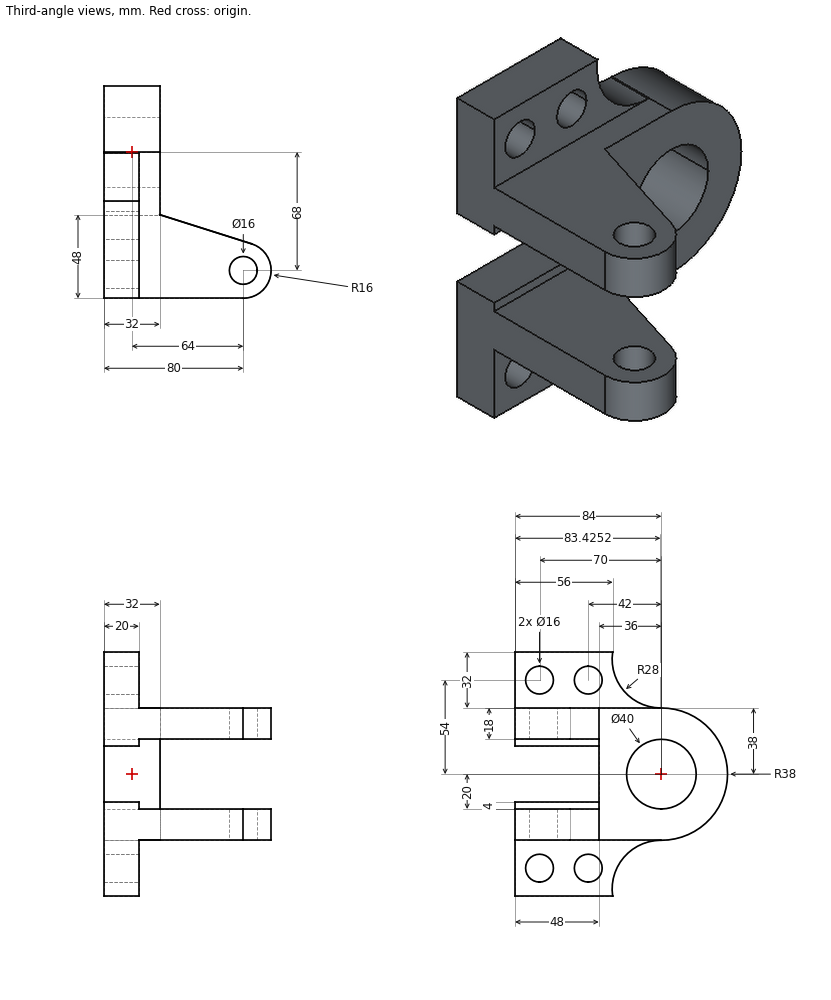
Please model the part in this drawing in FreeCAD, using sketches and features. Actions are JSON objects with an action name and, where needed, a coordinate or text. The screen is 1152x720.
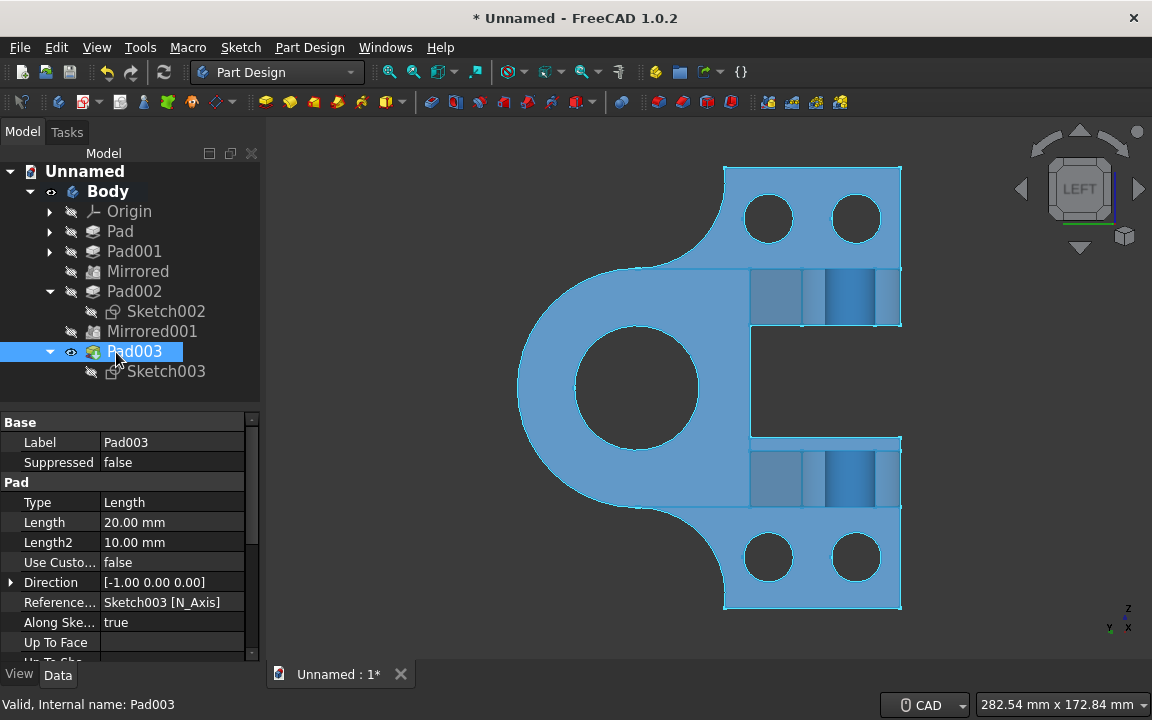
{"action": "left_click", "coordinate": [768, 102]}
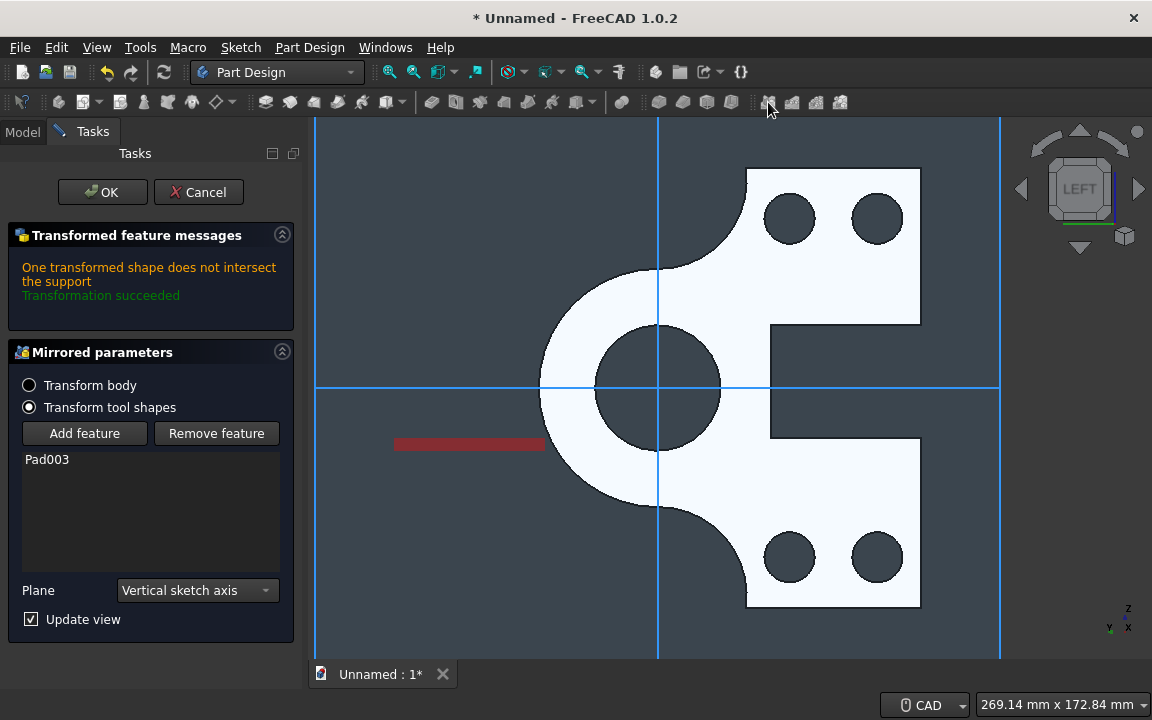
{"action": "left_click", "coordinate": [198, 590]}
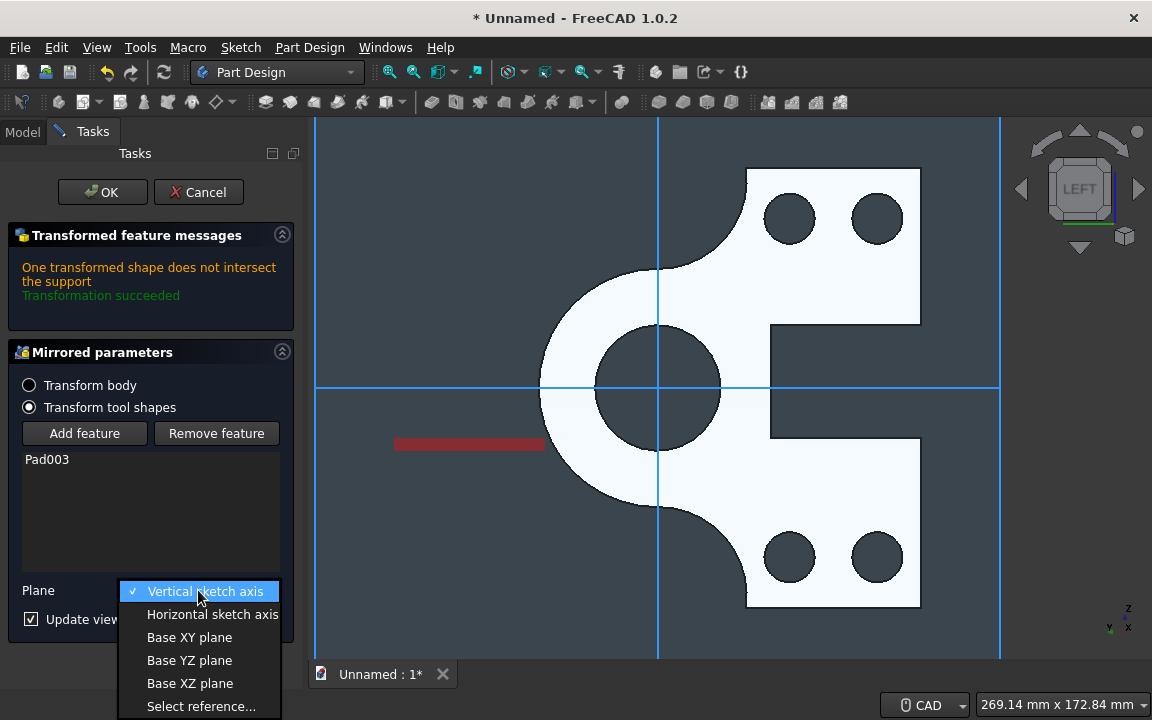
{"action": "left_click", "coordinate": [198, 638]}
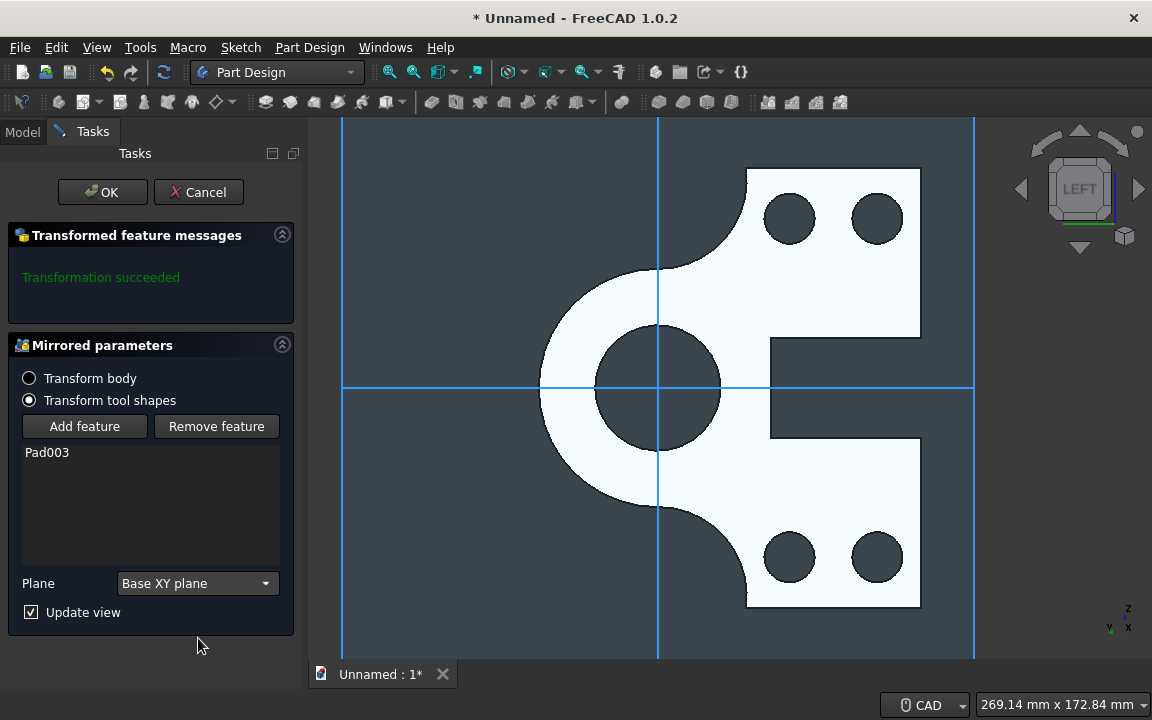
{"action": "left_click", "coordinate": [103, 192]}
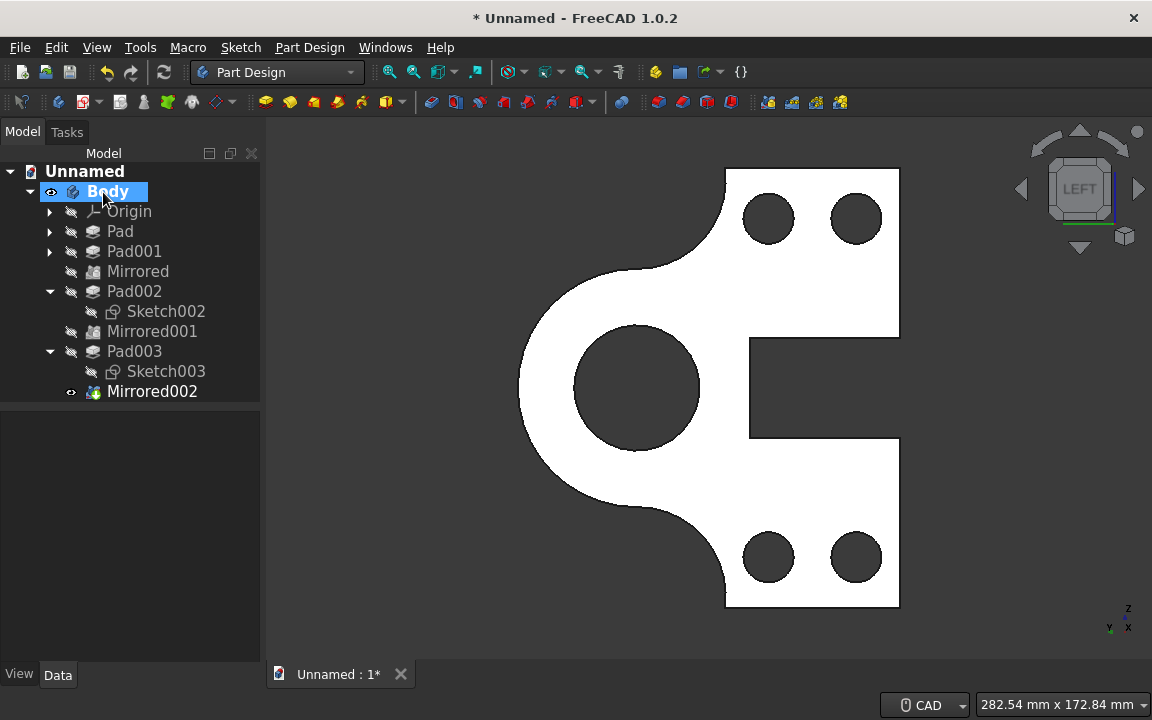
{"action": "key", "text": "0"}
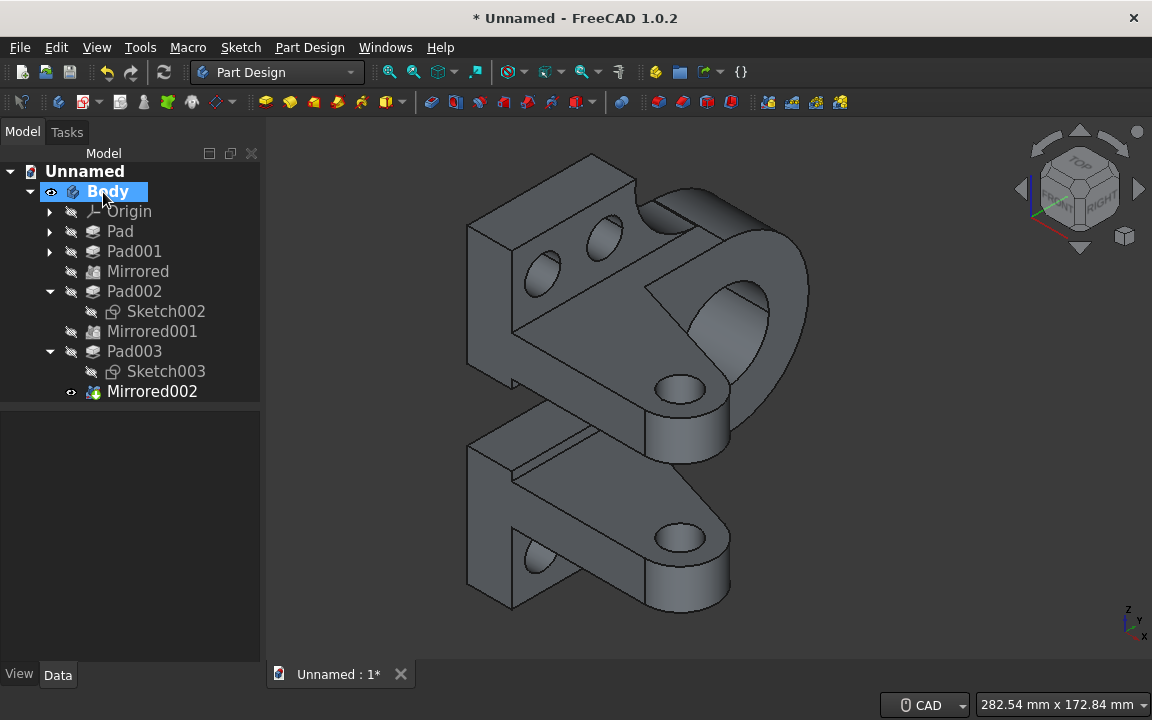
{"action": "key", "text": "v f"}